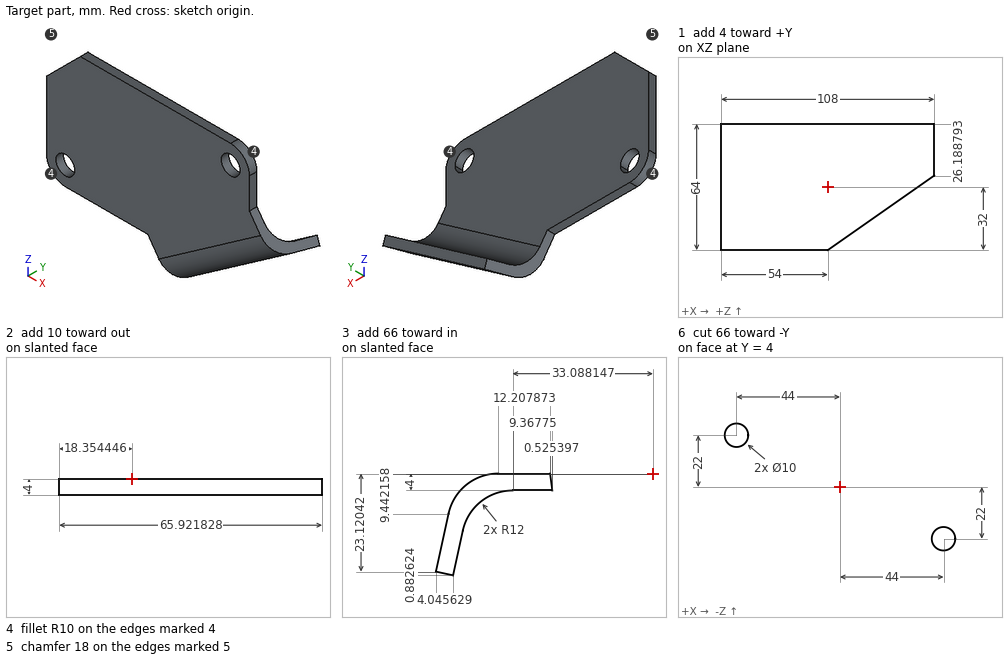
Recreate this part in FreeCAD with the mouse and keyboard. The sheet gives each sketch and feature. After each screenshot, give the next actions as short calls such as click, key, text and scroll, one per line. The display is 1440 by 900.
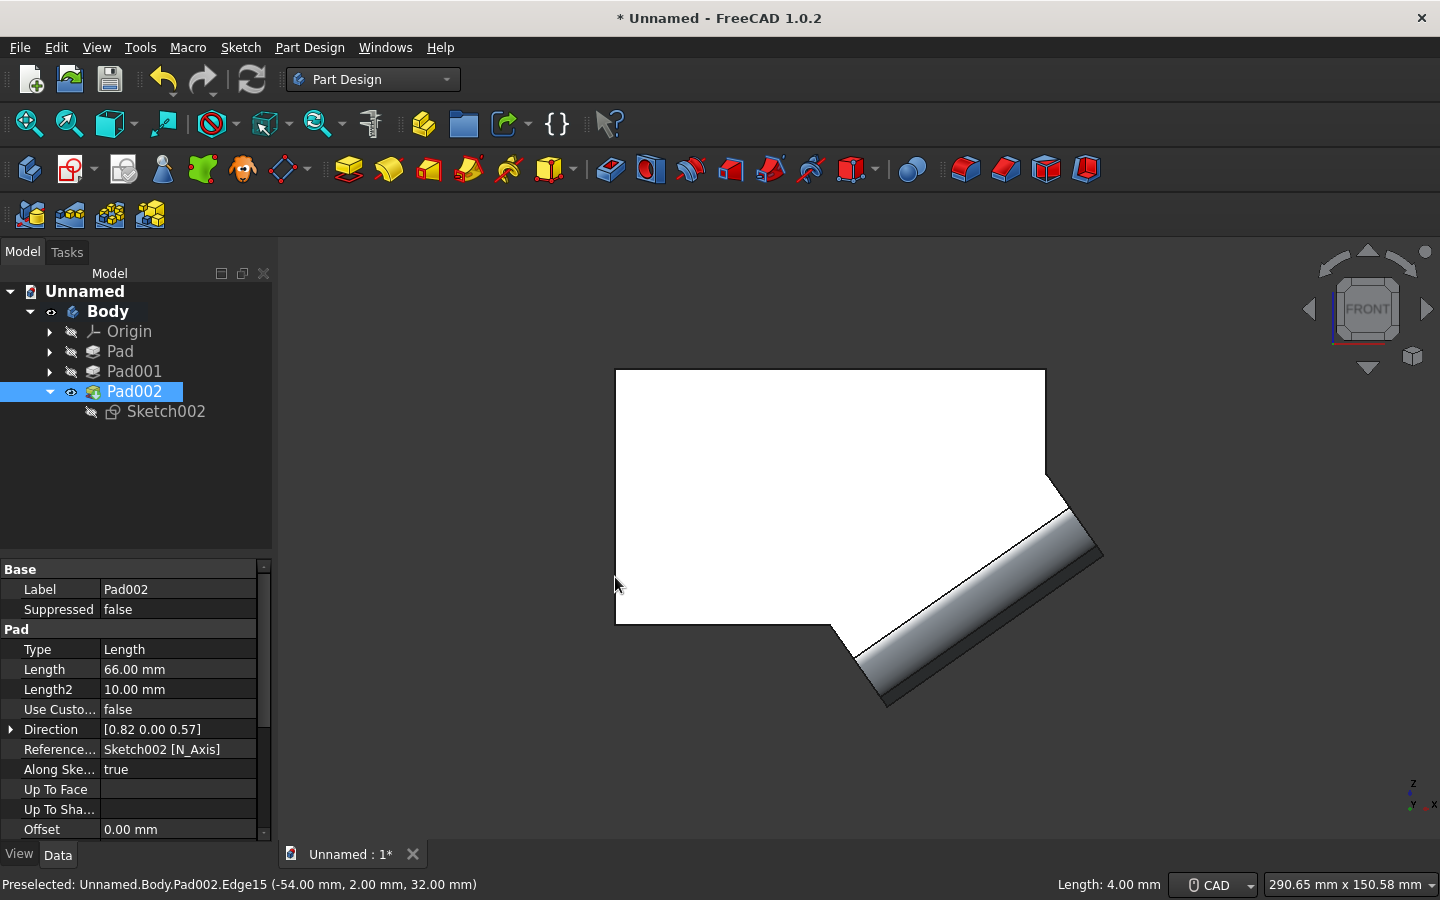
scroll(615, 624, up, 5)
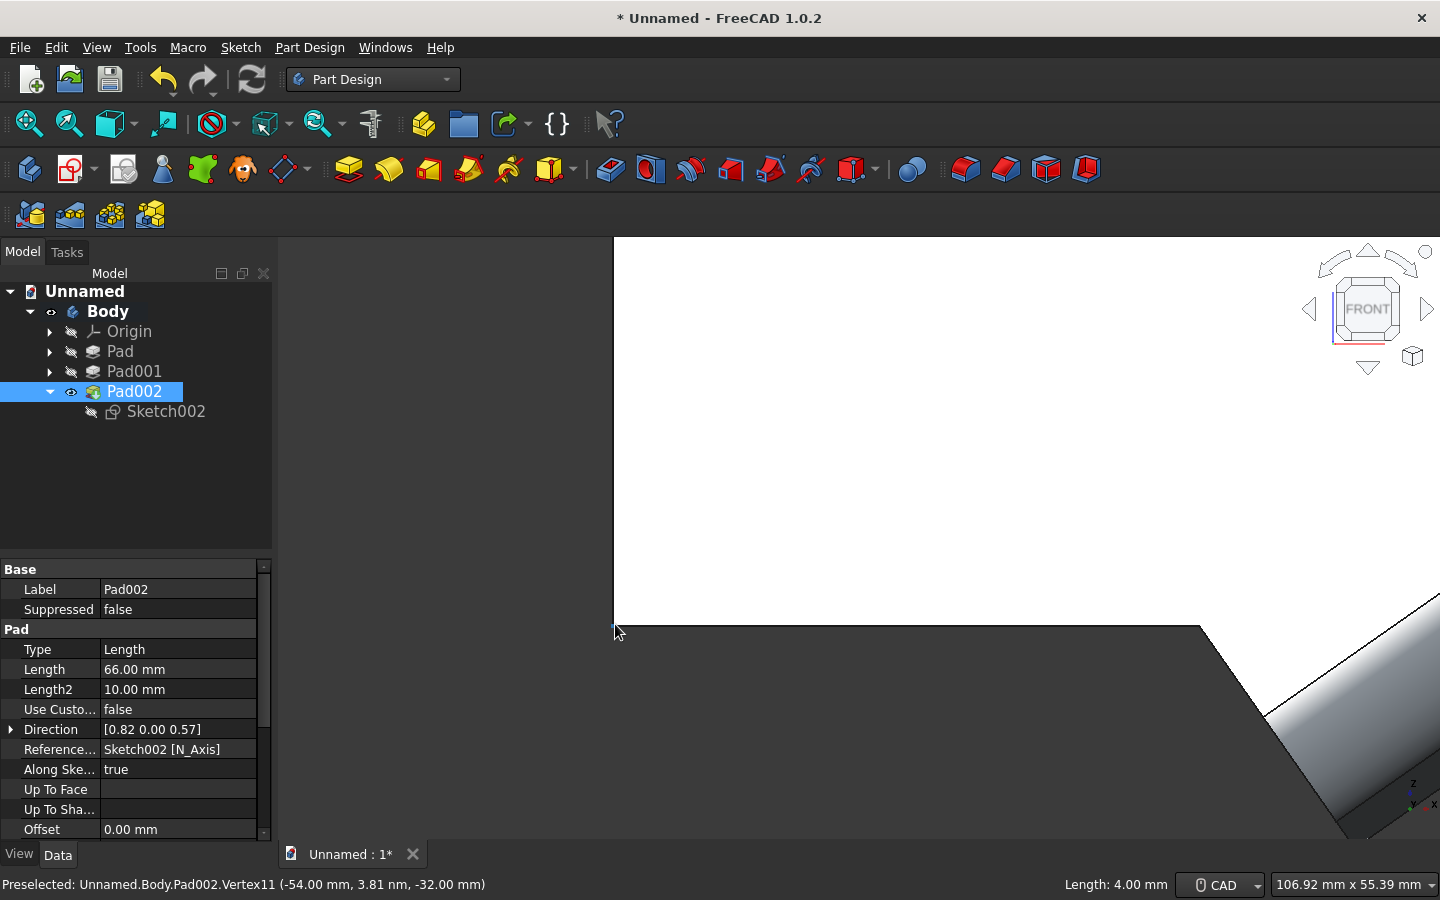
key(v)
key(f)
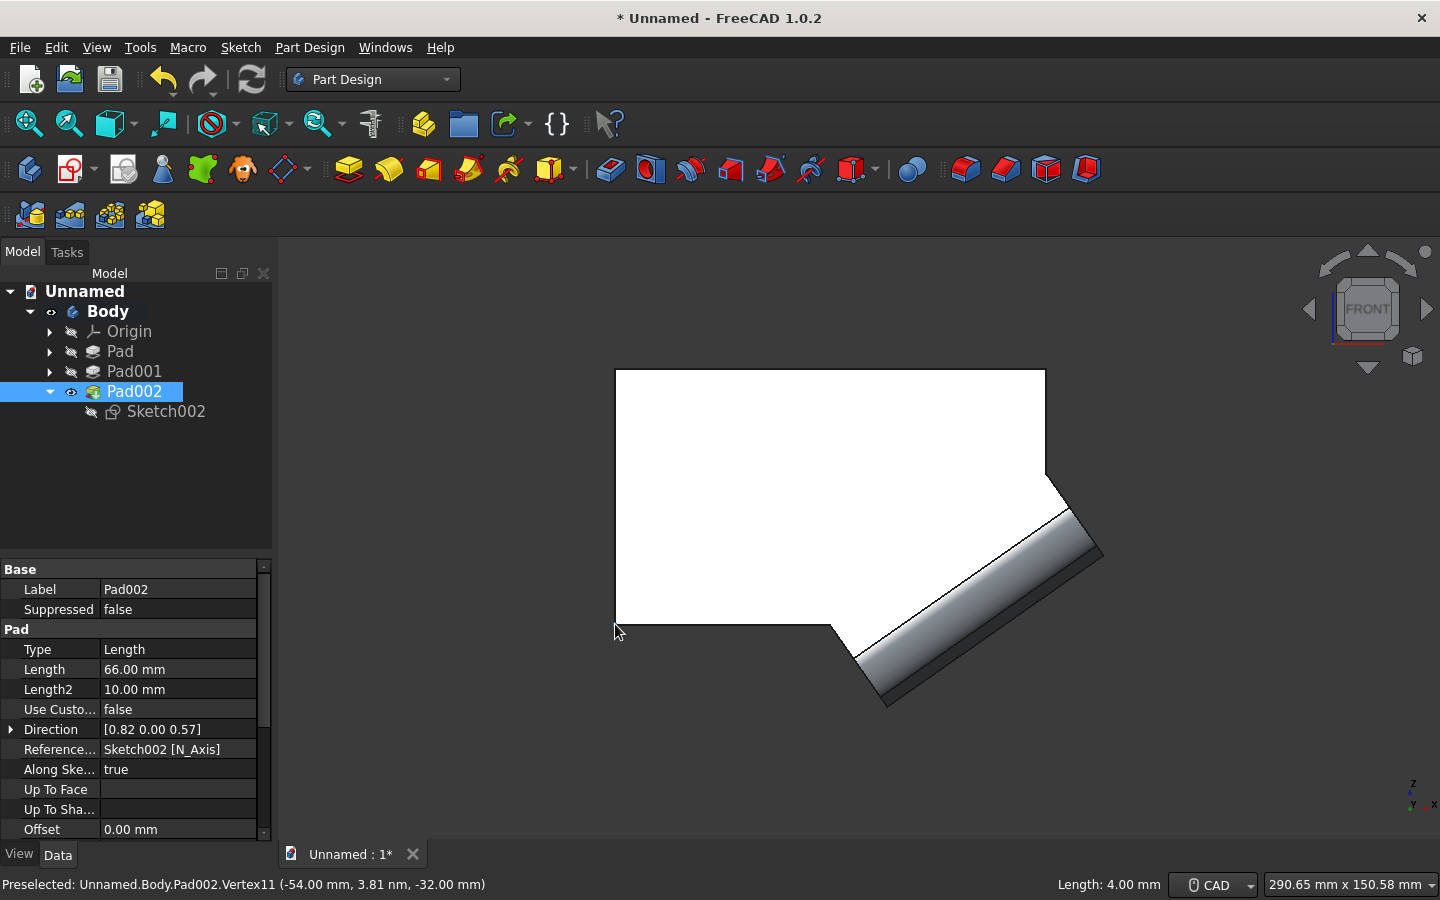
key(3)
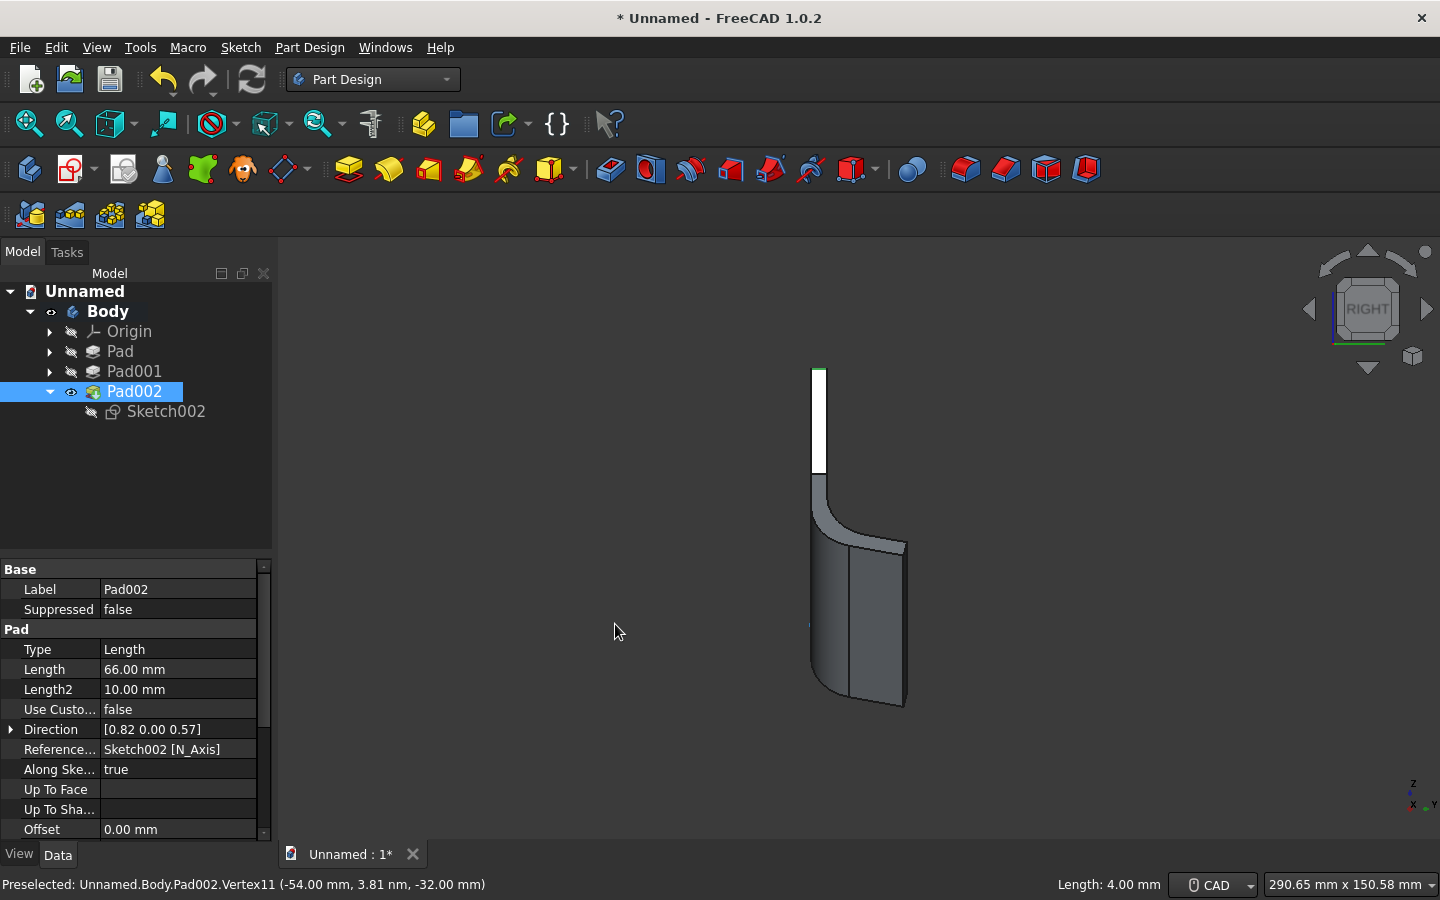
scroll(819, 624, up, 5)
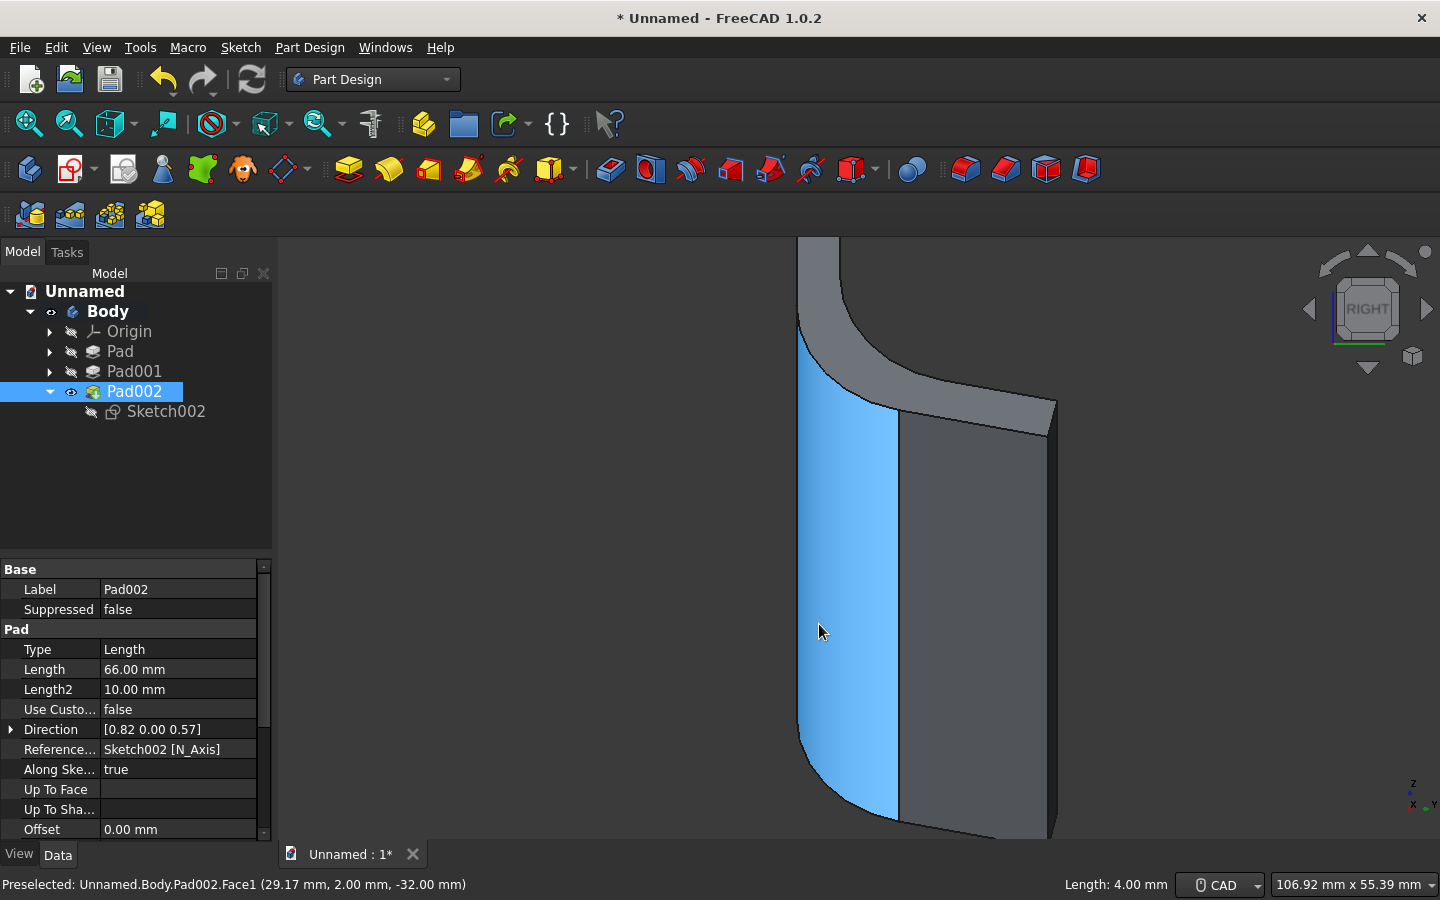
key(v)
key(f)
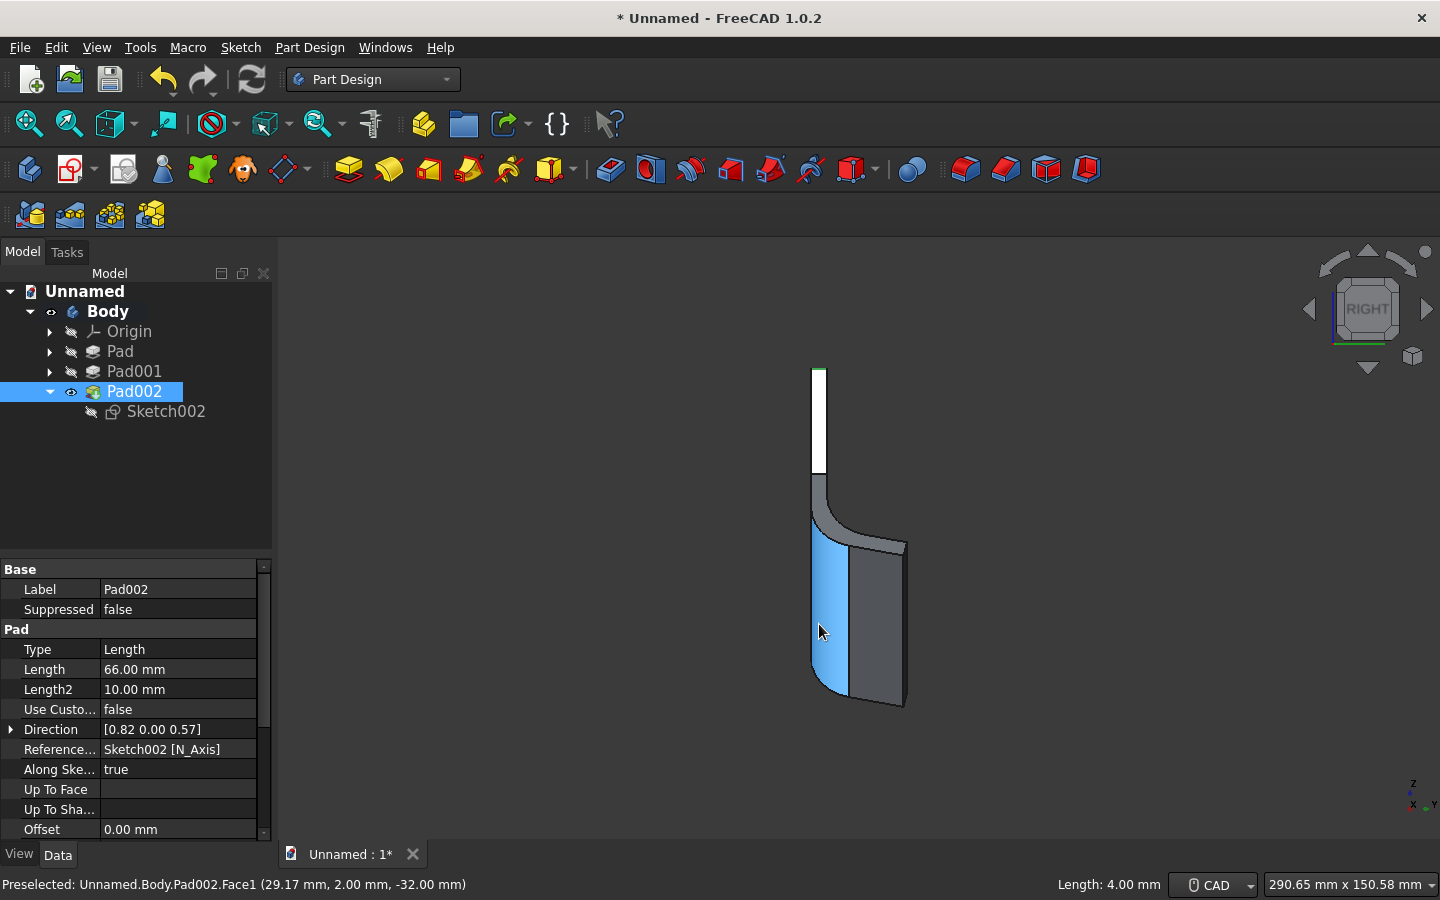
key(5)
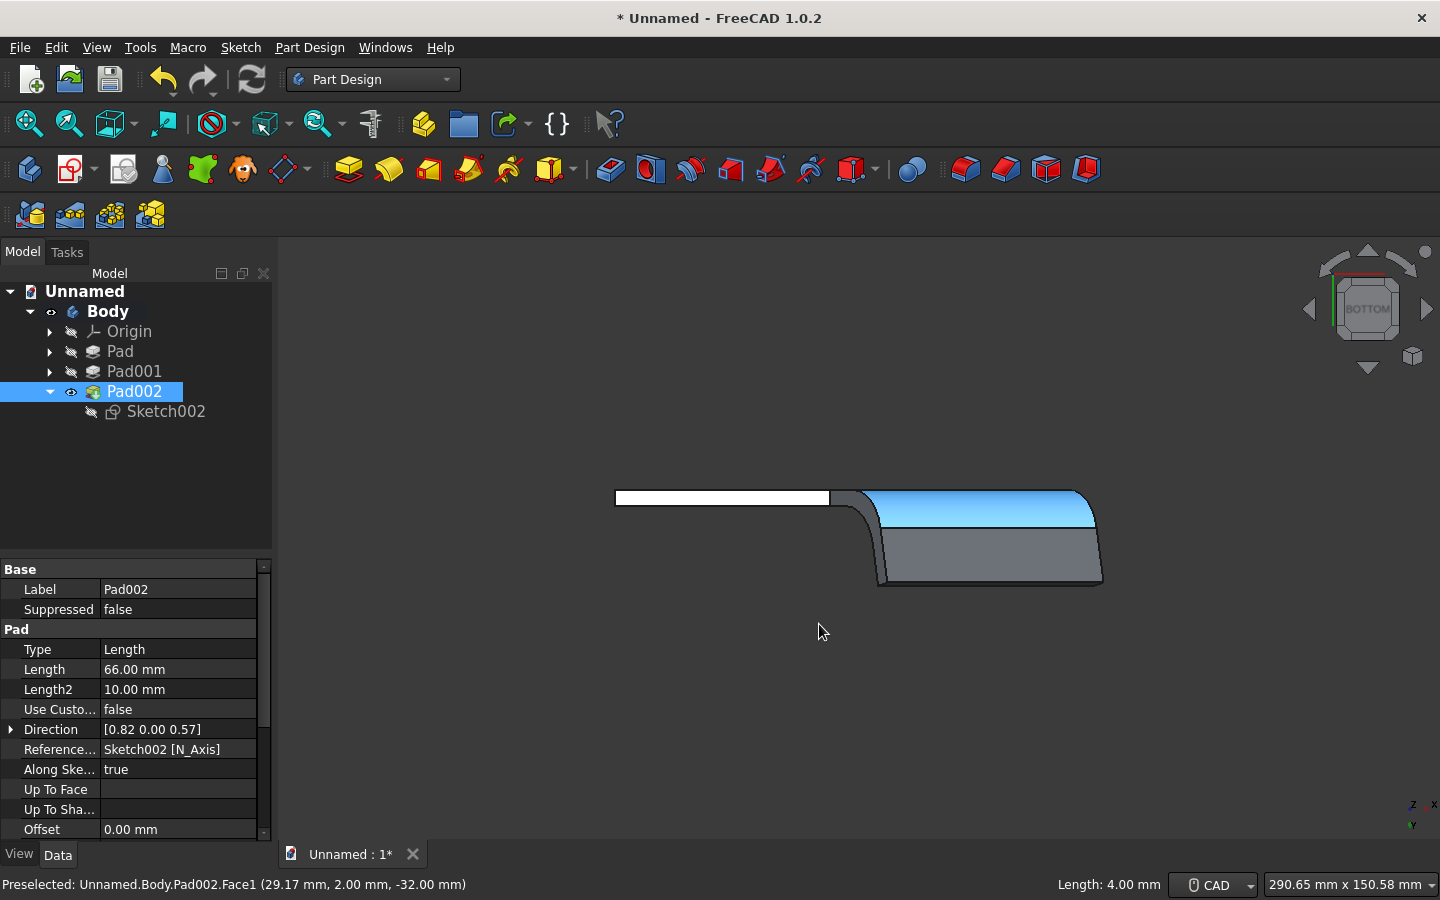
key(v)
key(f)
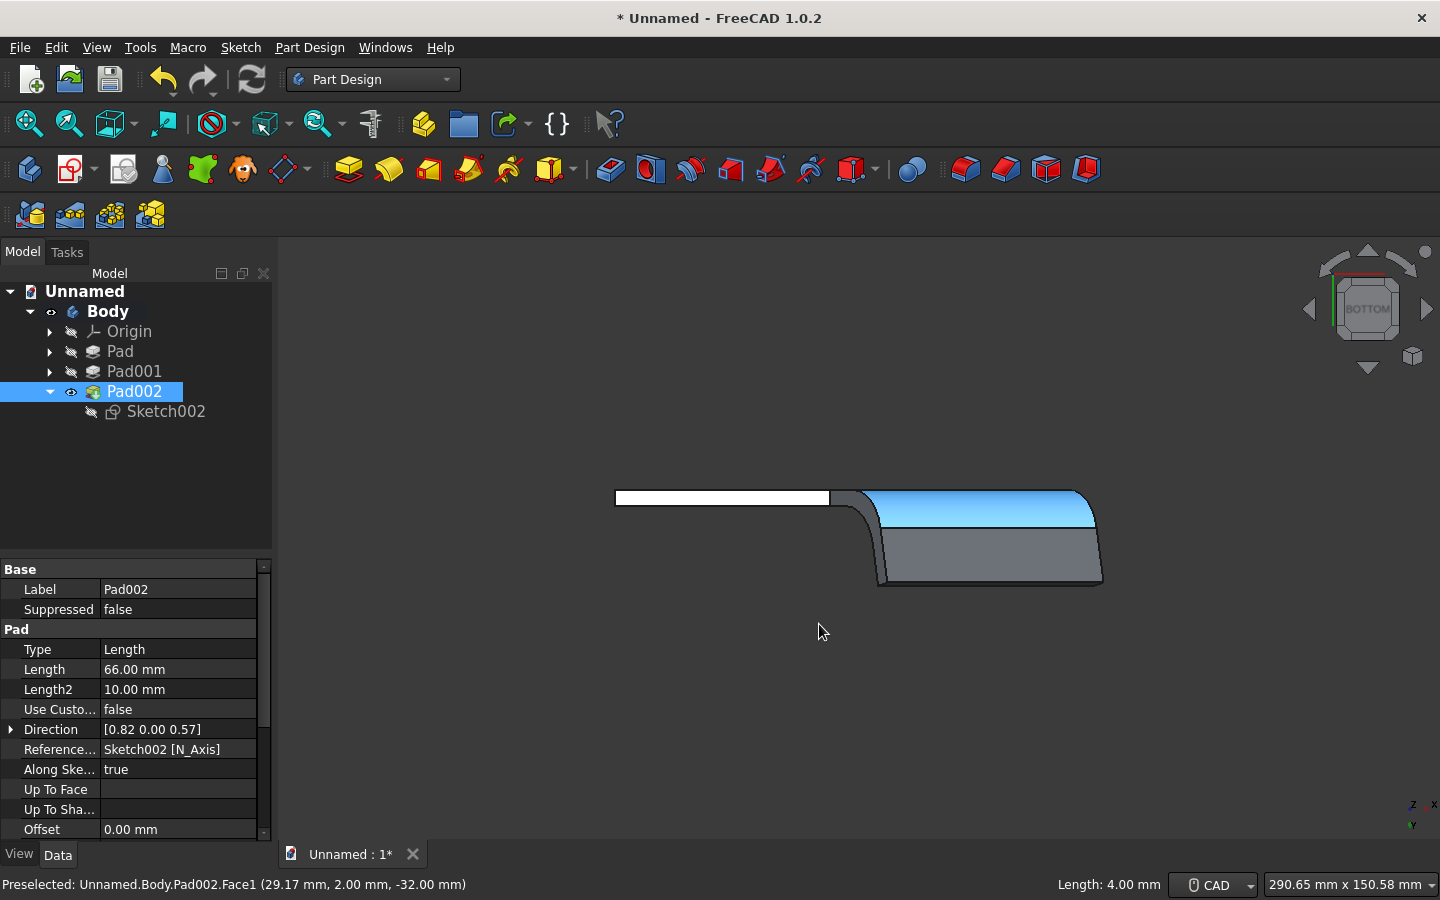
click(615, 497, ctrl)